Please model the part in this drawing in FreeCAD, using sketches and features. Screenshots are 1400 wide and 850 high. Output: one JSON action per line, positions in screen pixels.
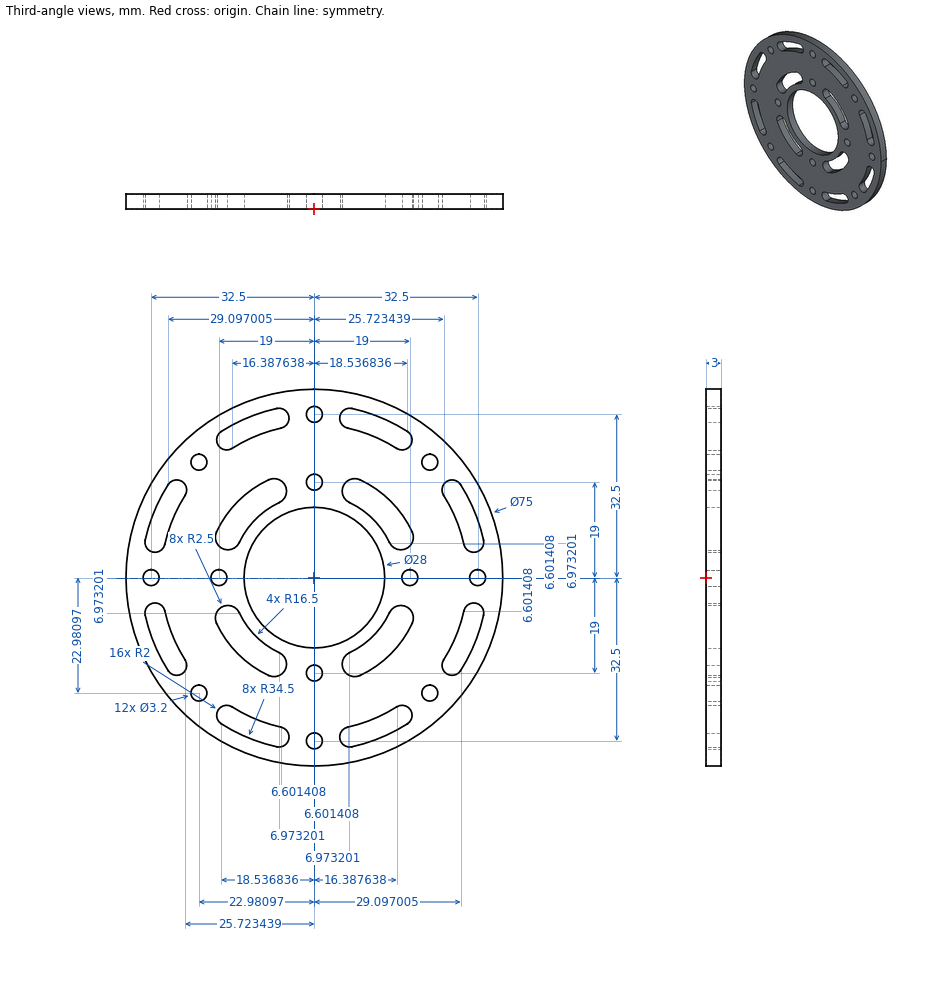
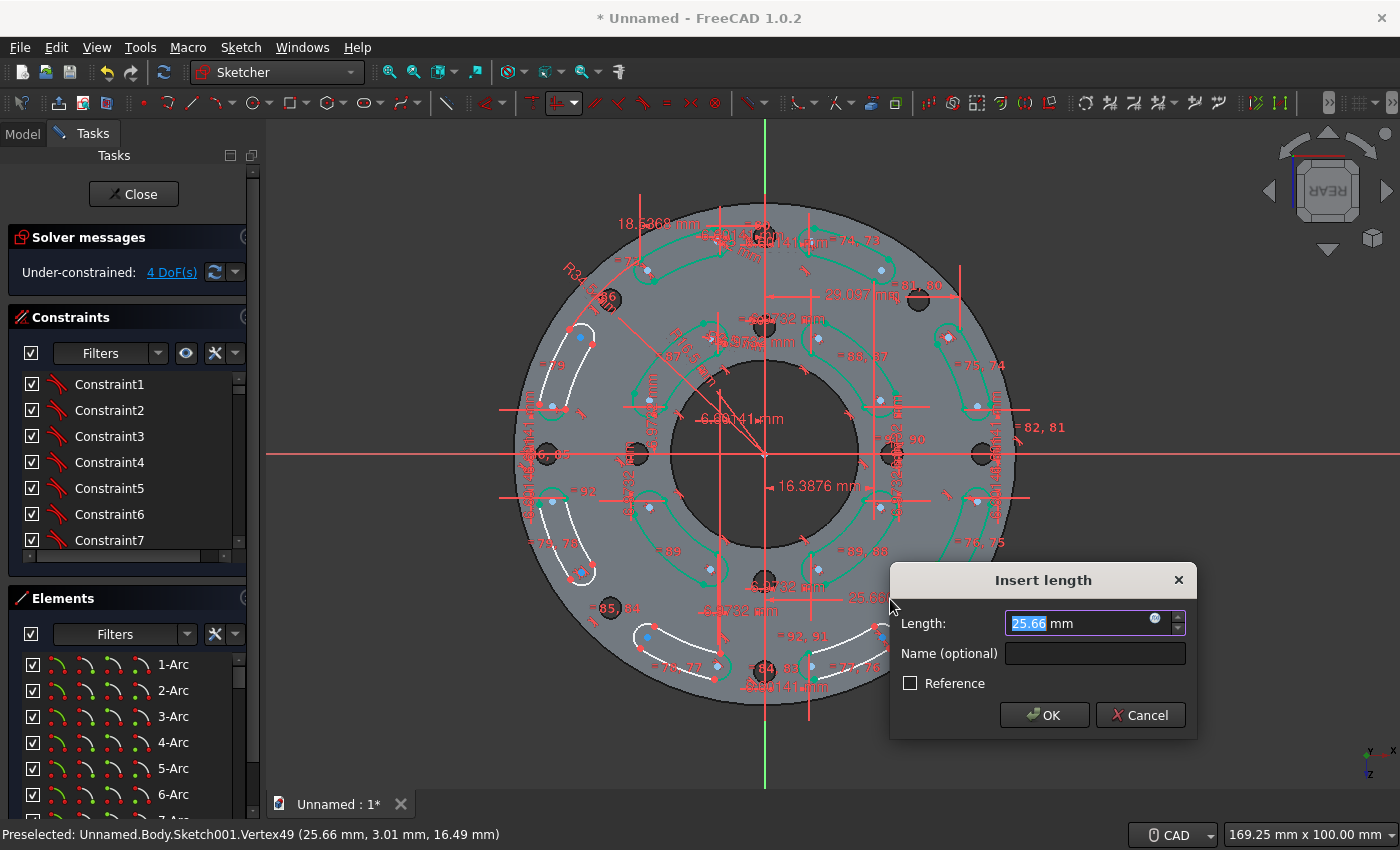
{"action": "type", "text": "25.723439"}
{"action": "key", "text": "Return"}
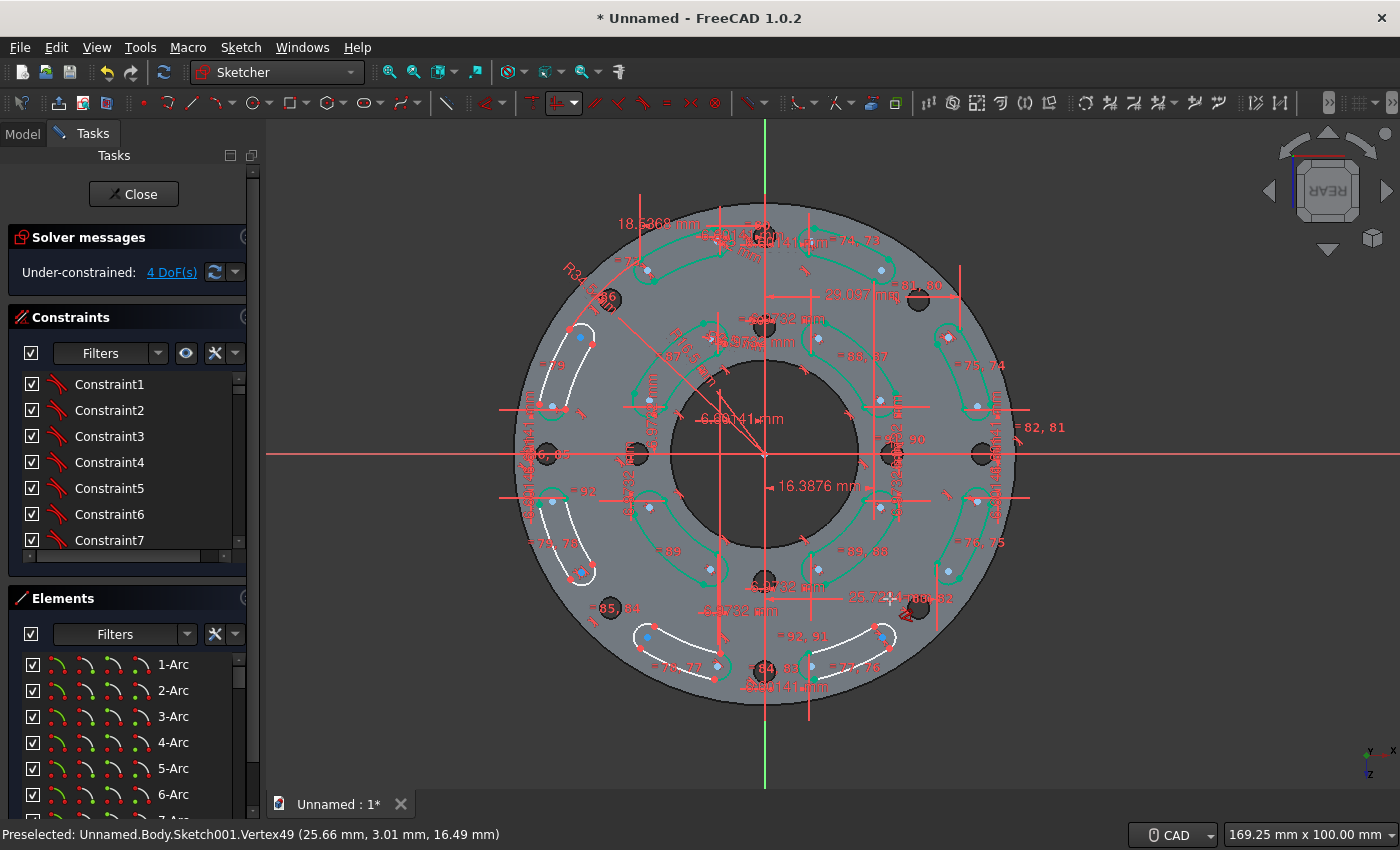
{"action": "left_click", "coordinate": [889, 649]}
{"action": "left_click", "coordinate": [871, 683]}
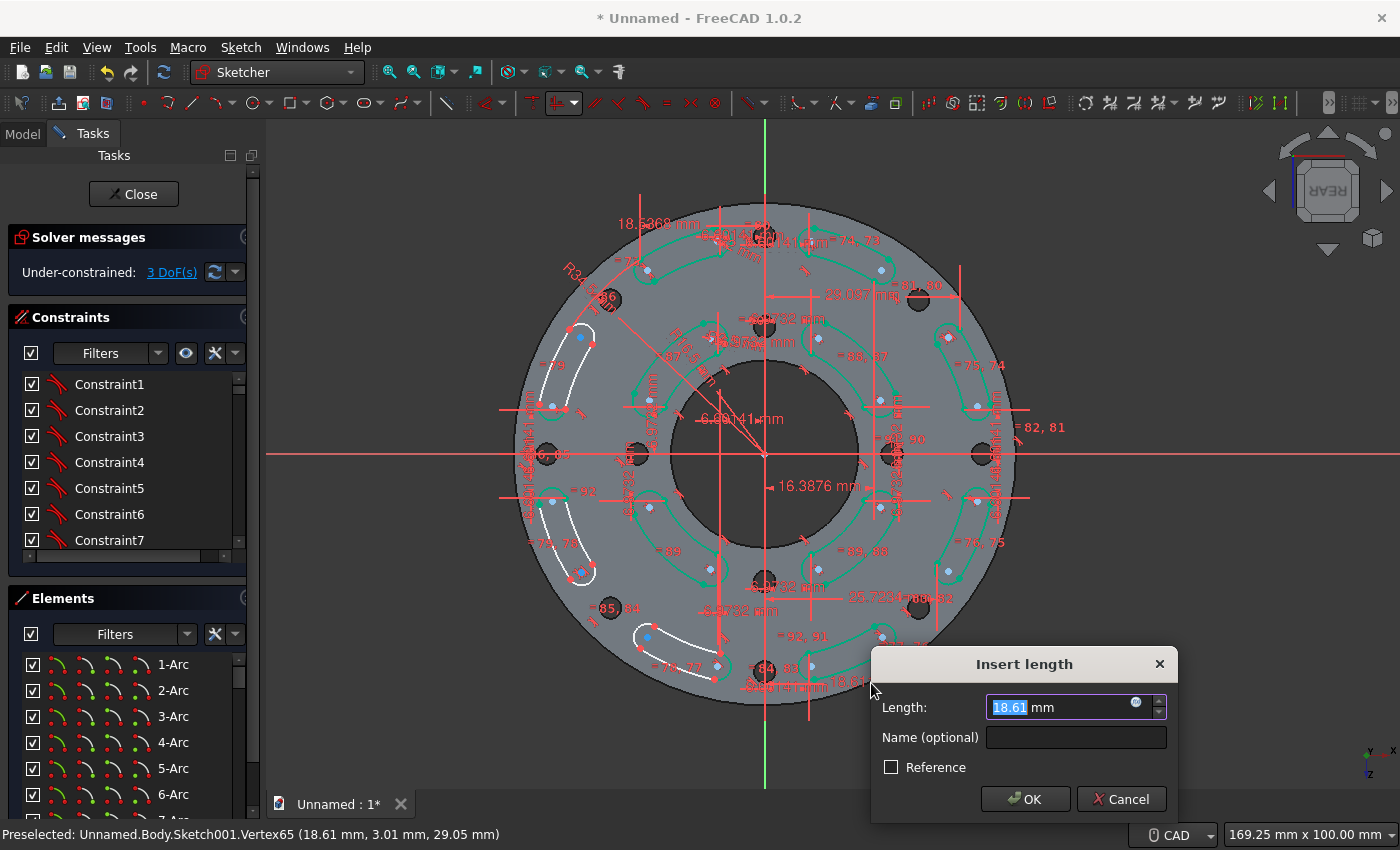
{"action": "type", "text": "18.536836"}
{"action": "key", "text": "Return"}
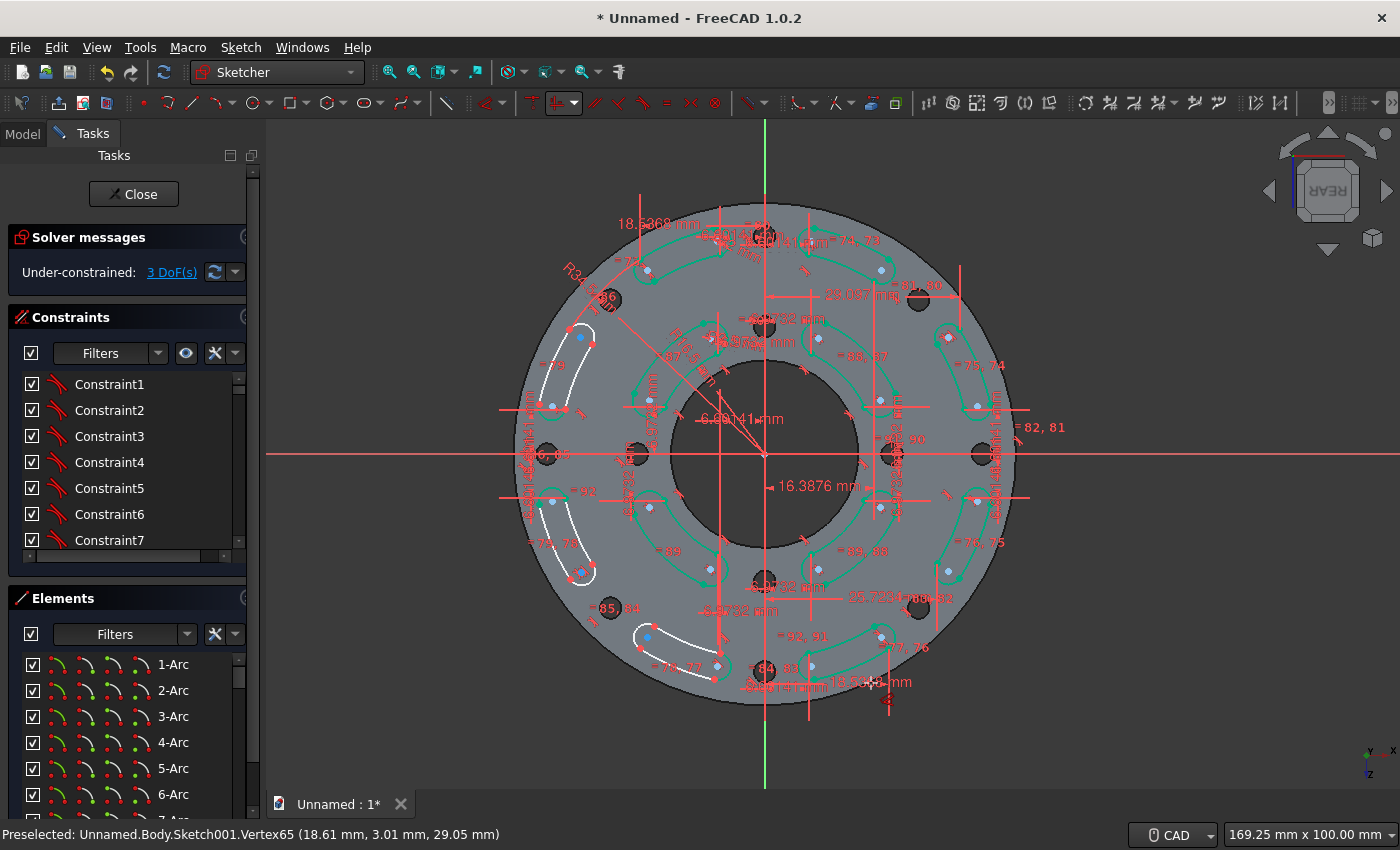
{"action": "left_click", "coordinate": [654, 626]}
{"action": "left_click", "coordinate": [748, 660]}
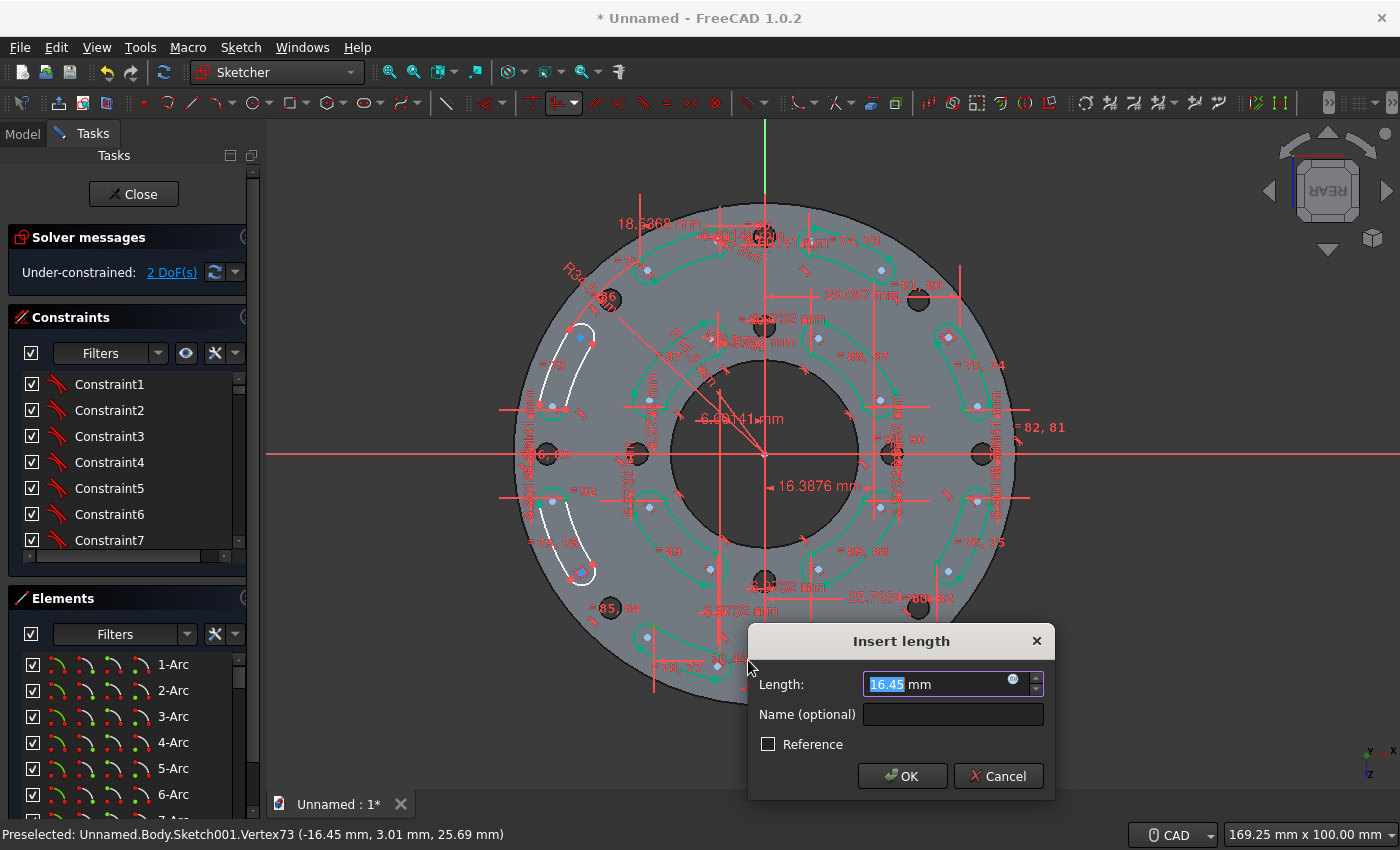
{"action": "type", "text": "16.387638"}
{"action": "key", "text": "Return"}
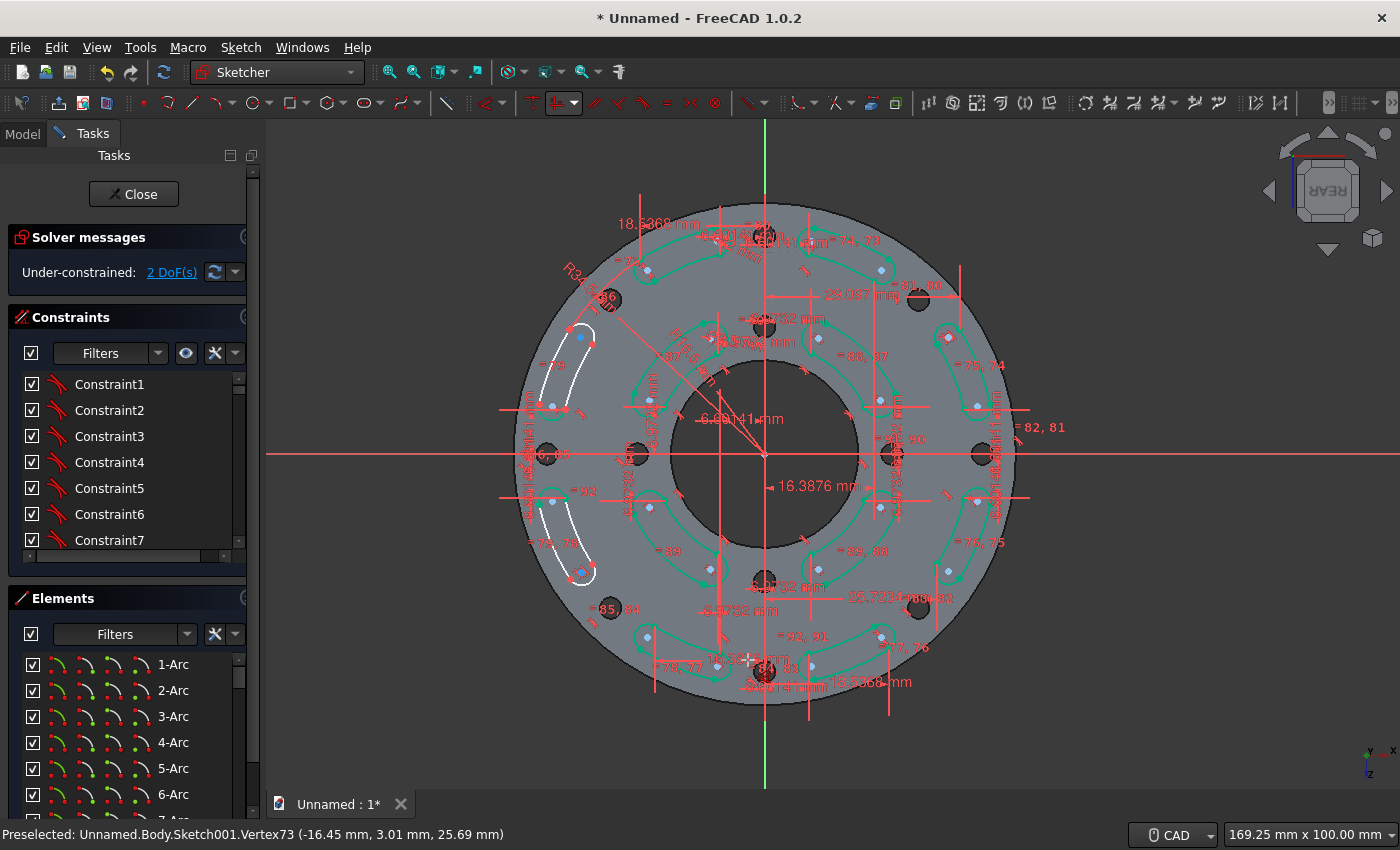
{"action": "left_click", "coordinate": [570, 579]}
{"action": "left_click", "coordinate": [668, 613]}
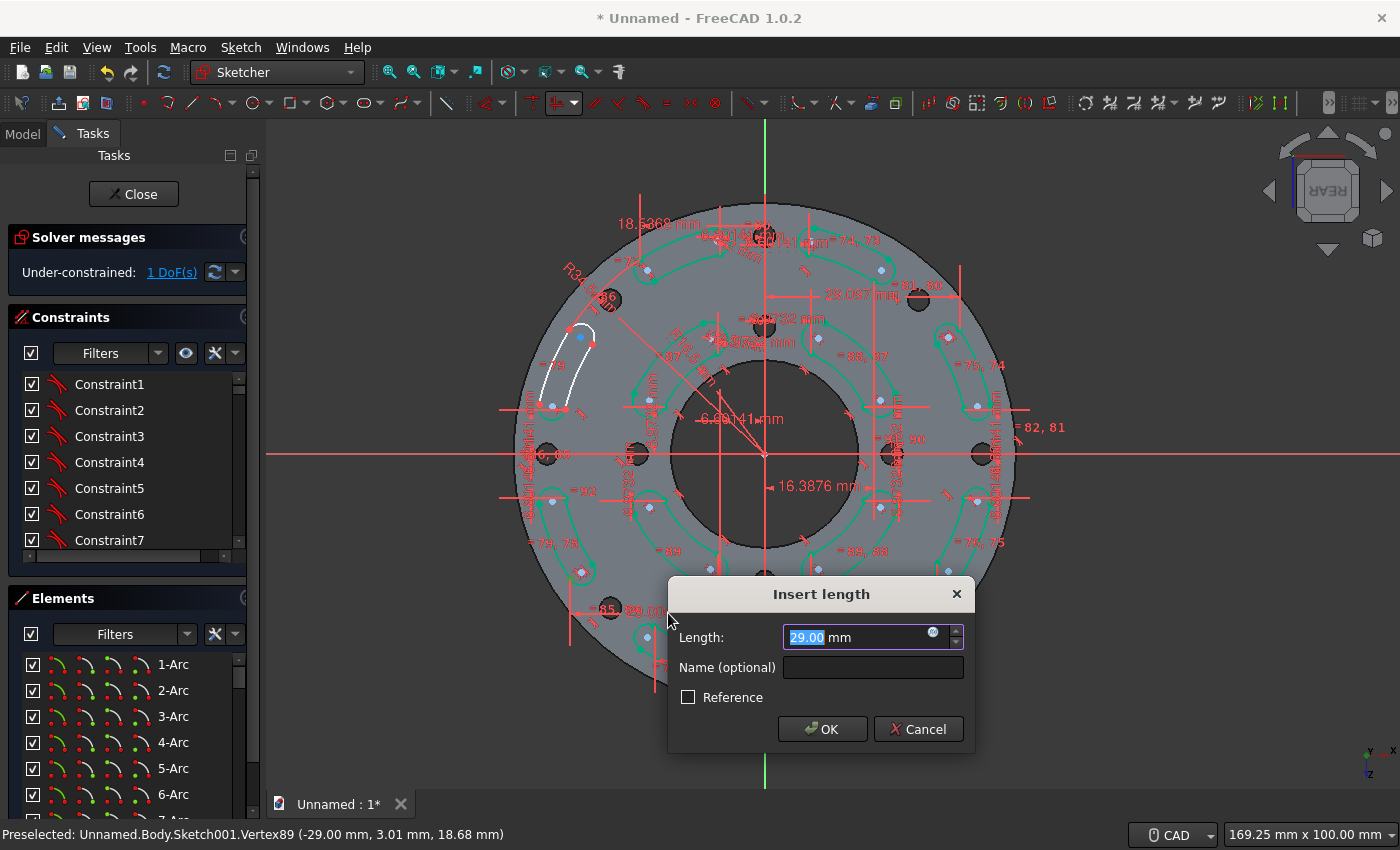
{"action": "type", "text": "29.097005"}
{"action": "key", "text": "Return"}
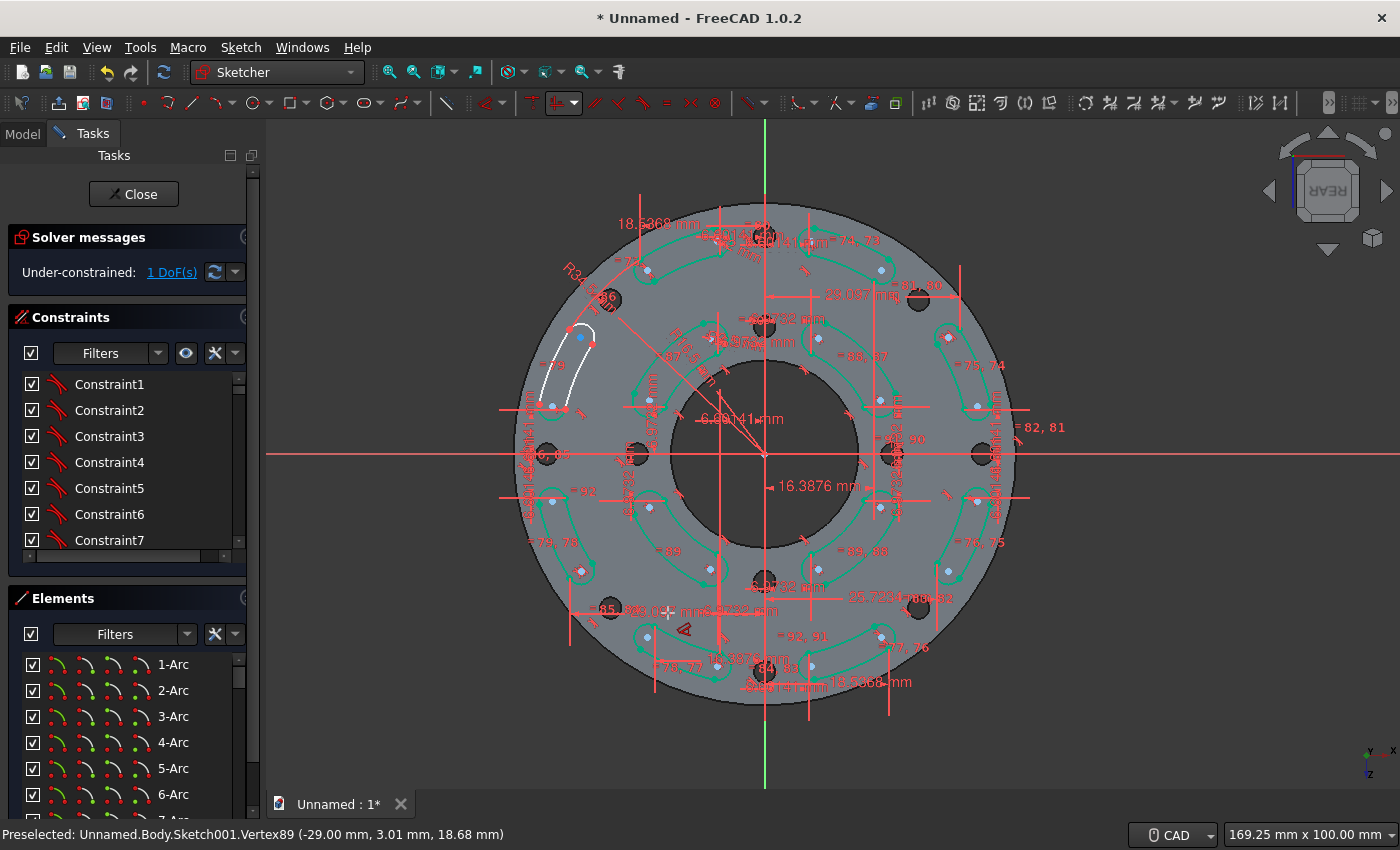
{"action": "left_click", "coordinate": [592, 344]}
{"action": "left_click", "coordinate": [678, 310]}